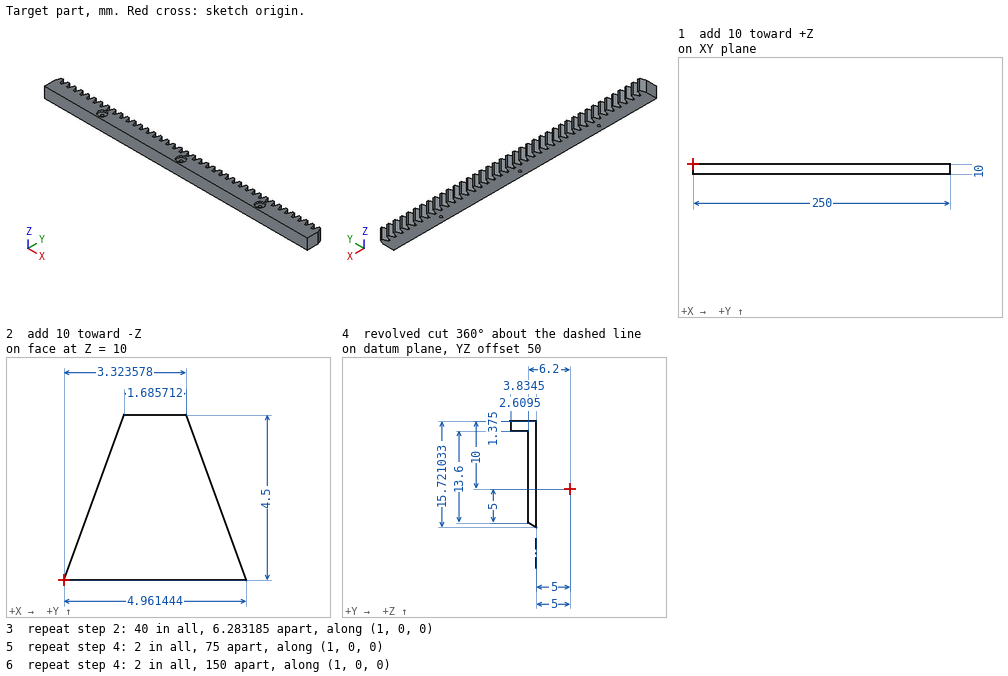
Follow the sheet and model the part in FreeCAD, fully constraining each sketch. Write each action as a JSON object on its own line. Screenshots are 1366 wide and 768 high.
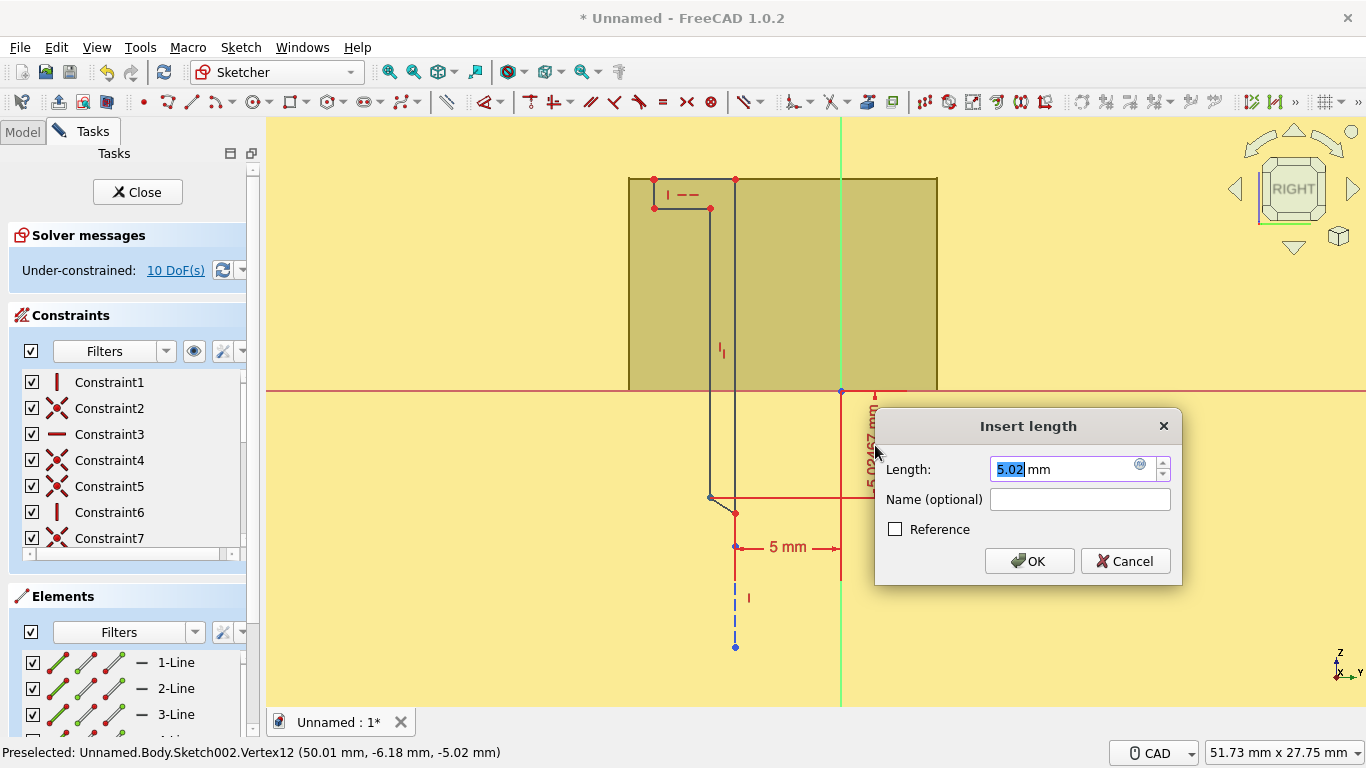
{"action": "type", "text": "5"}
{"action": "key", "text": "Return"}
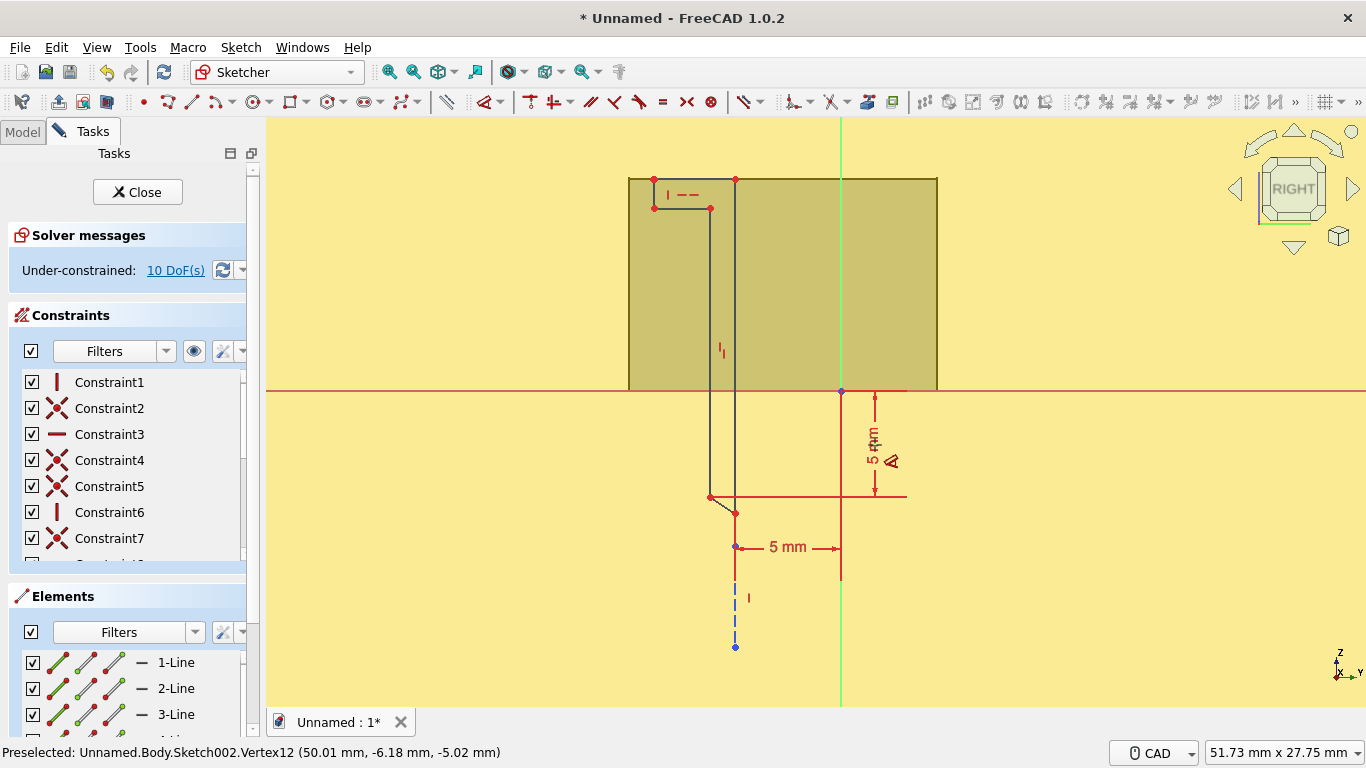
{"action": "left_click", "coordinate": [735, 547]}
{"action": "left_click", "coordinate": [788, 581]}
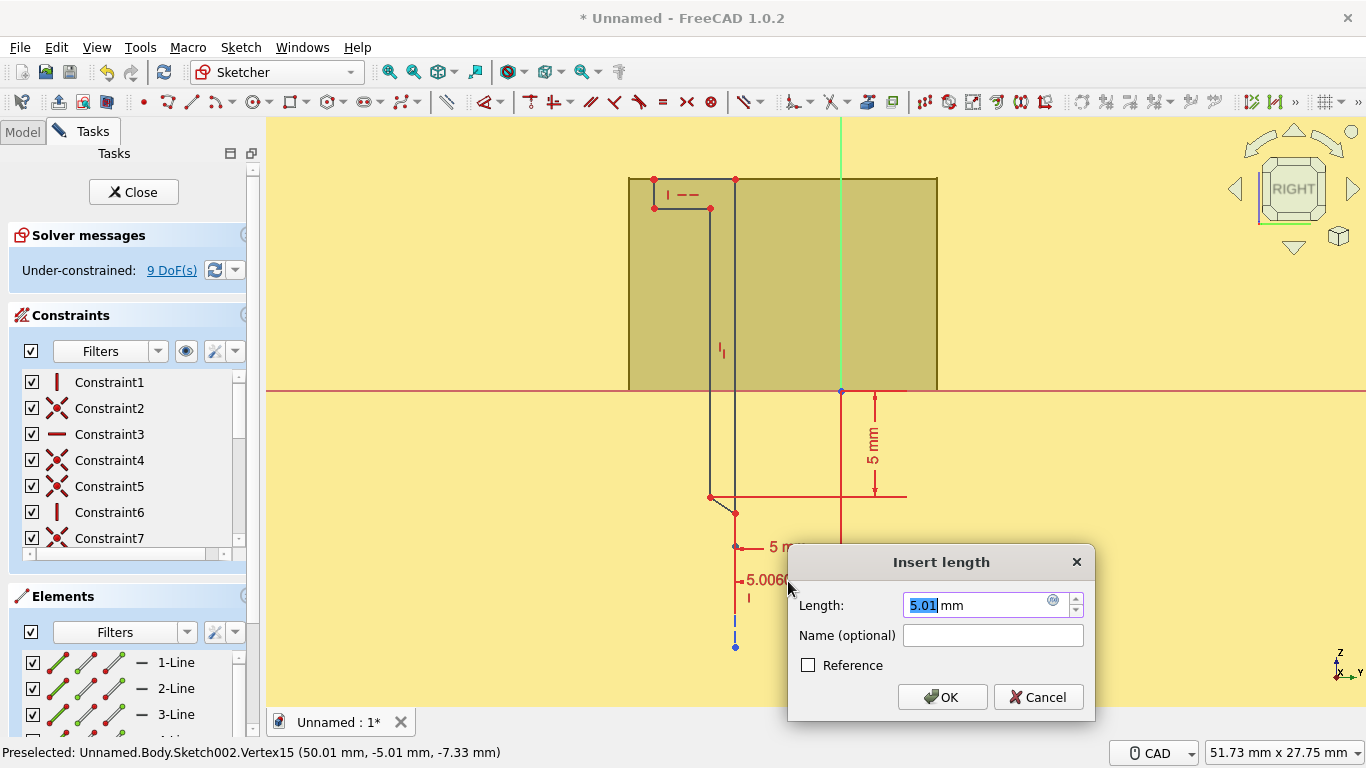
{"action": "type", "text": "5"}
{"action": "key", "text": "Return"}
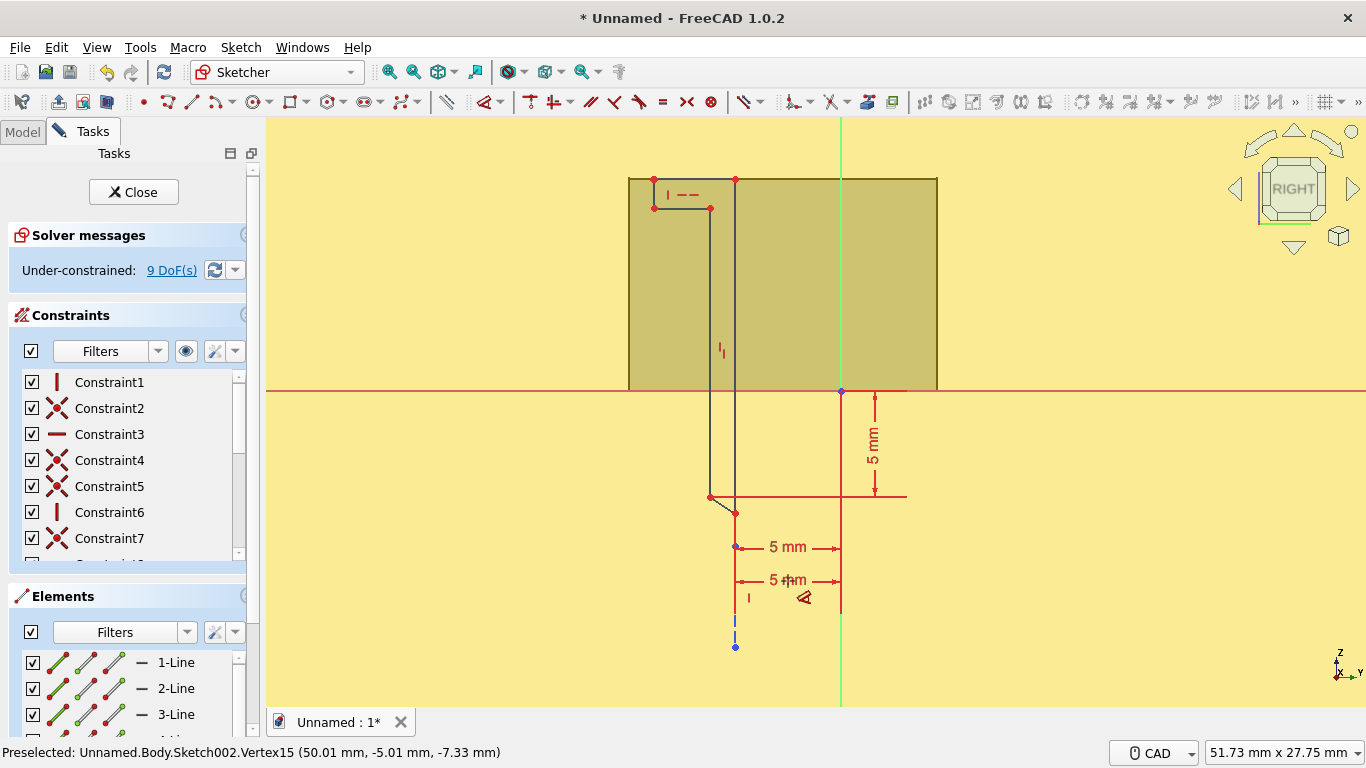
{"action": "left_click", "coordinate": [735, 179]}
{"action": "left_click", "coordinate": [875, 285]}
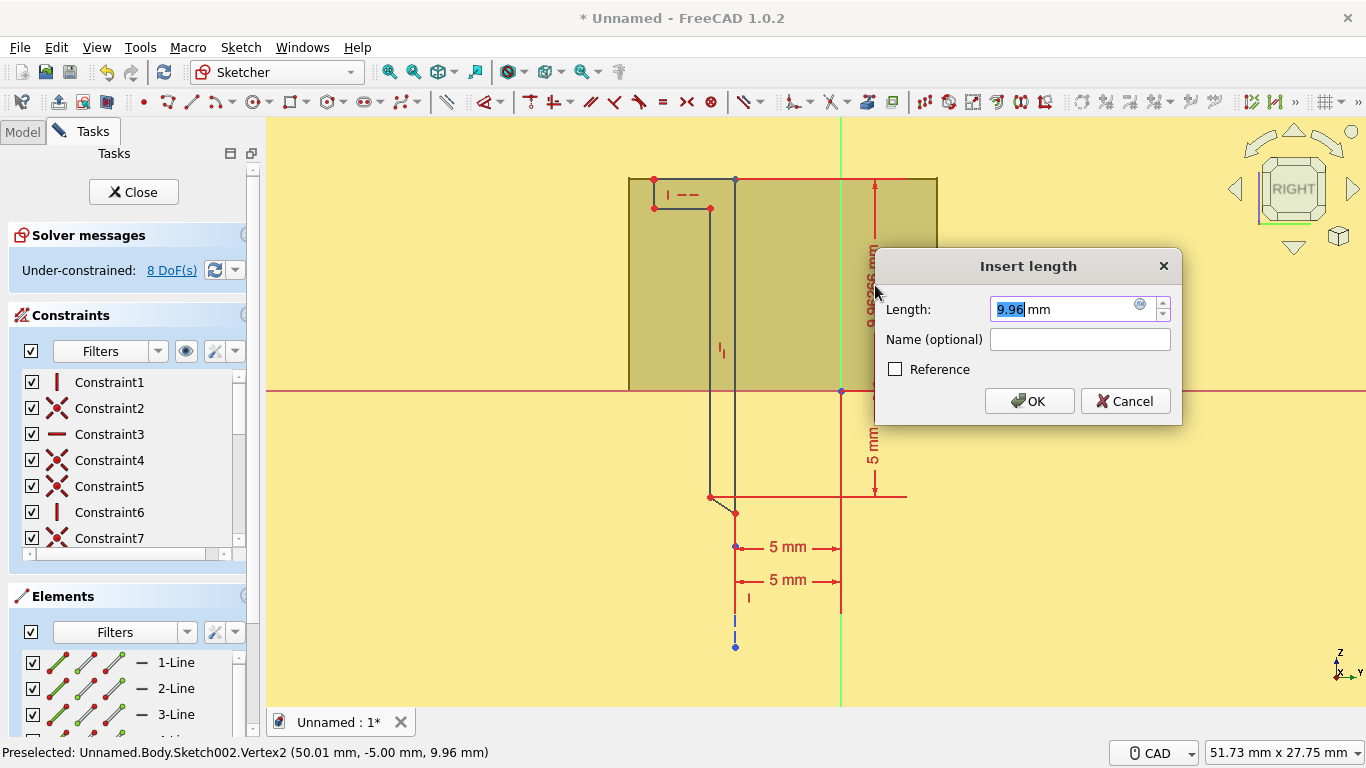
{"action": "type", "text": "10"}
{"action": "key", "text": "Return"}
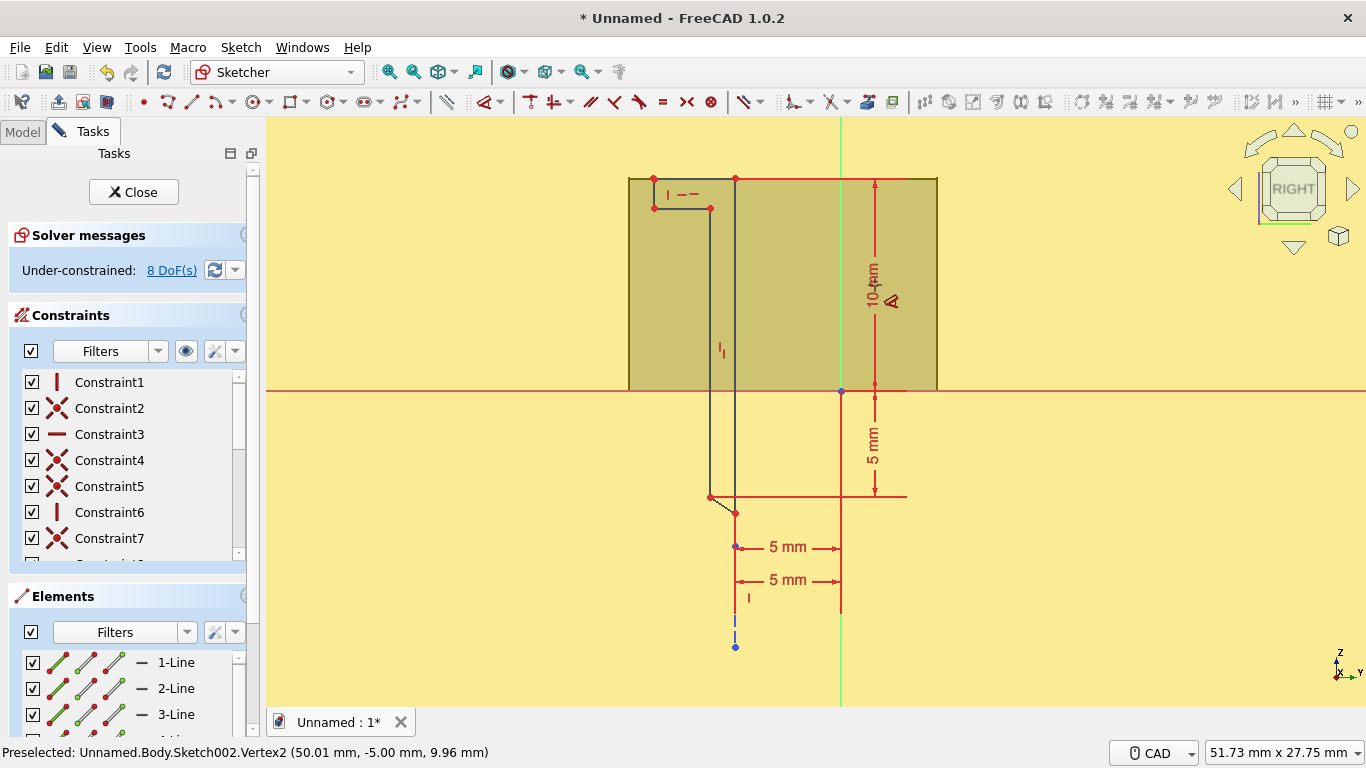
{"action": "left_click", "coordinate": [710, 296]}
{"action": "left_click", "coordinate": [676, 353]}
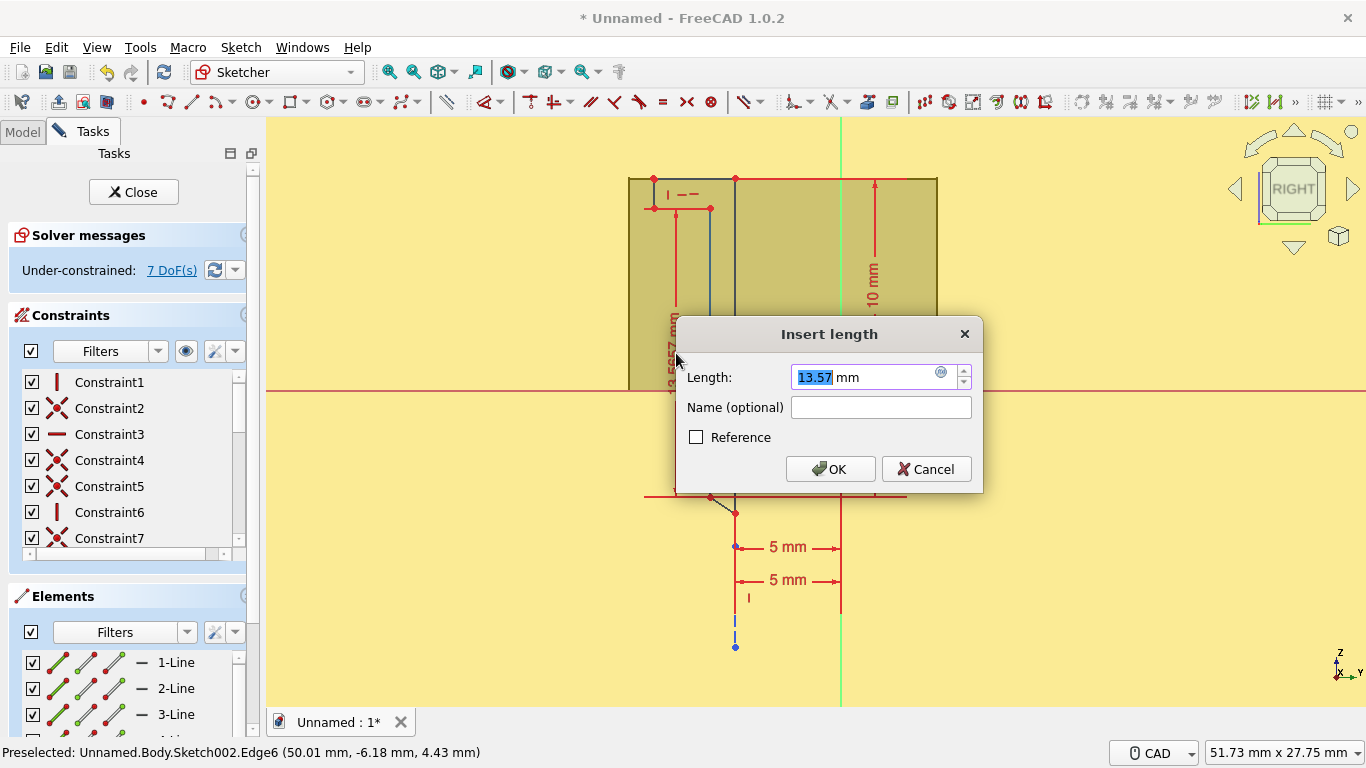
{"action": "type", "text": "13.6"}
{"action": "key", "text": "Return"}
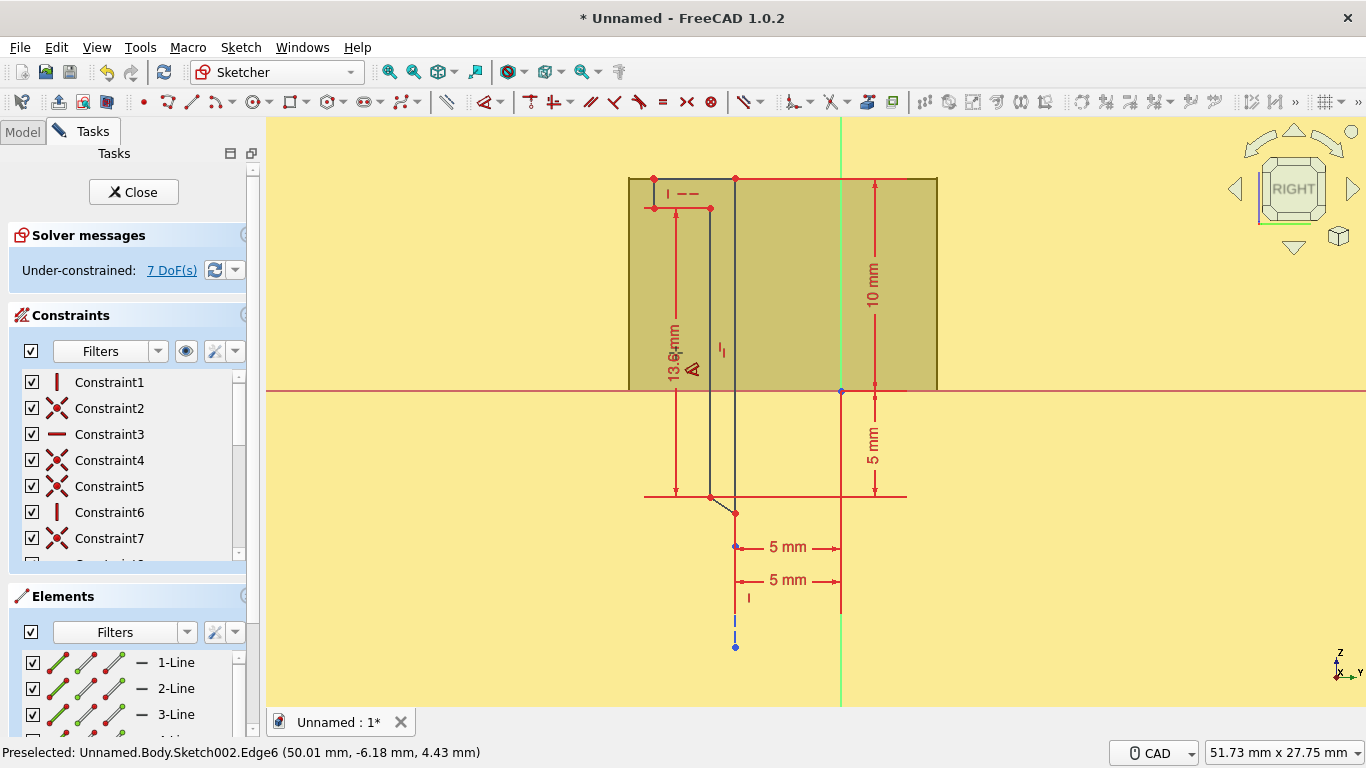
{"action": "left_click", "coordinate": [710, 208]}
{"action": "left_click", "coordinate": [776, 174]}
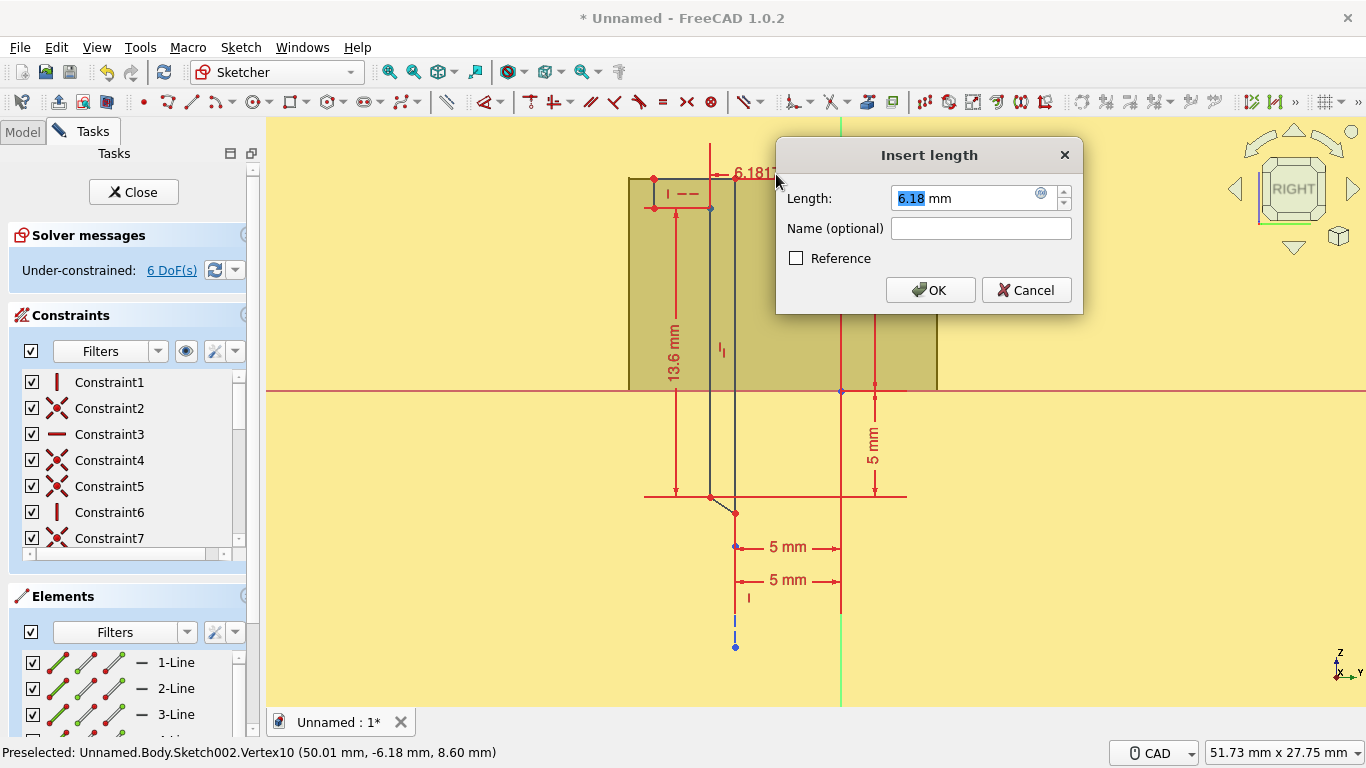
{"action": "type", "text": "6.2"}
{"action": "key", "text": "Return"}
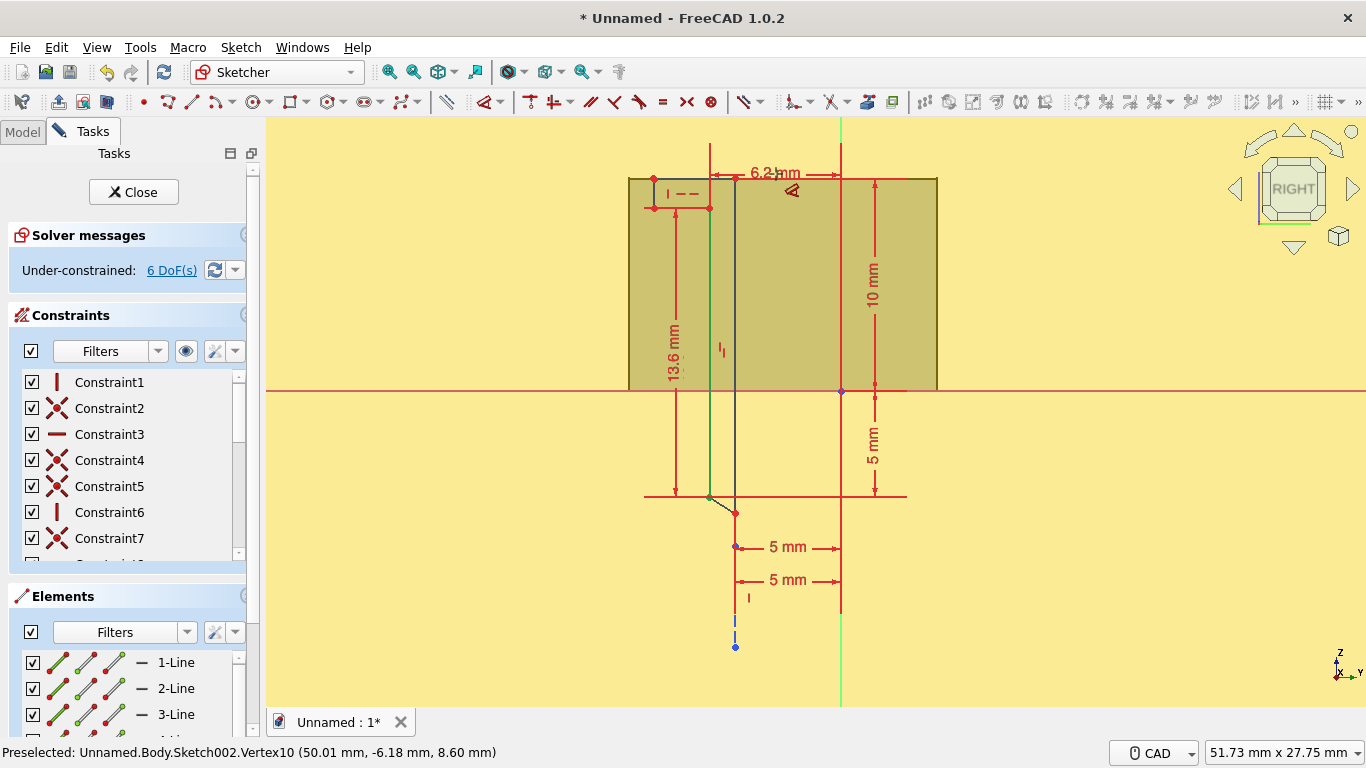
{"action": "scroll", "coordinate": [654, 191], "scroll_direction": "up", "scroll_amount": 2}